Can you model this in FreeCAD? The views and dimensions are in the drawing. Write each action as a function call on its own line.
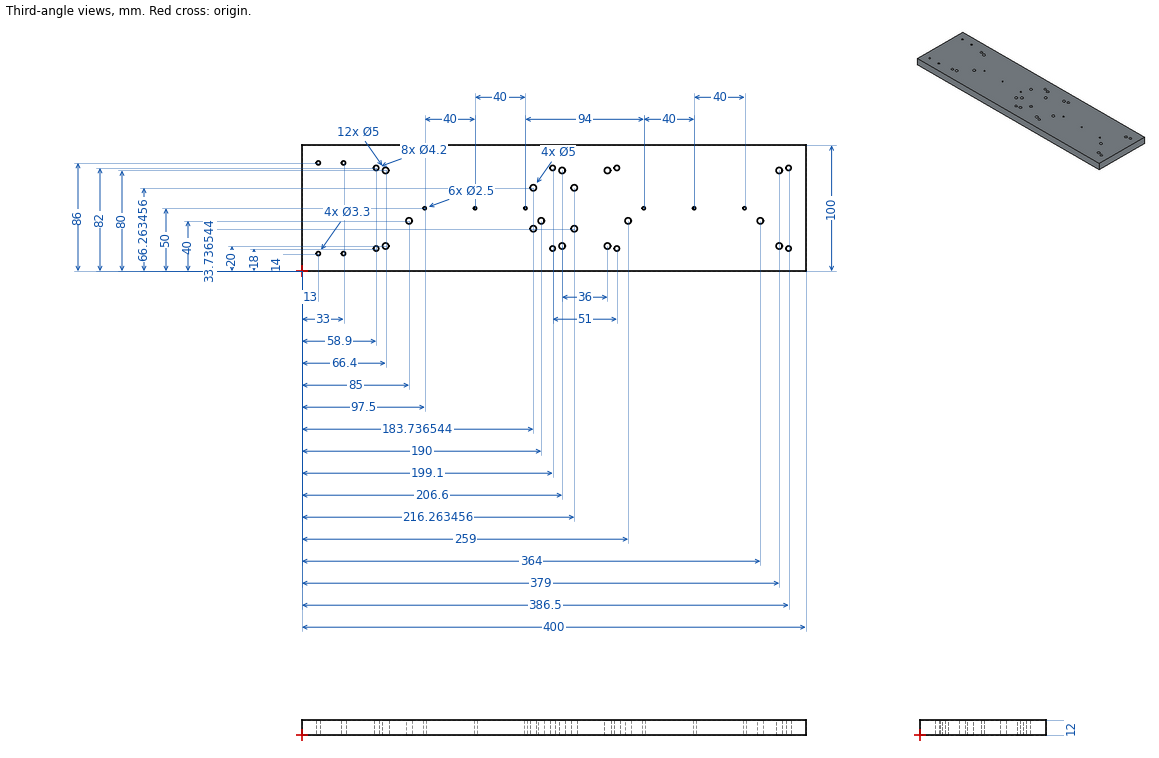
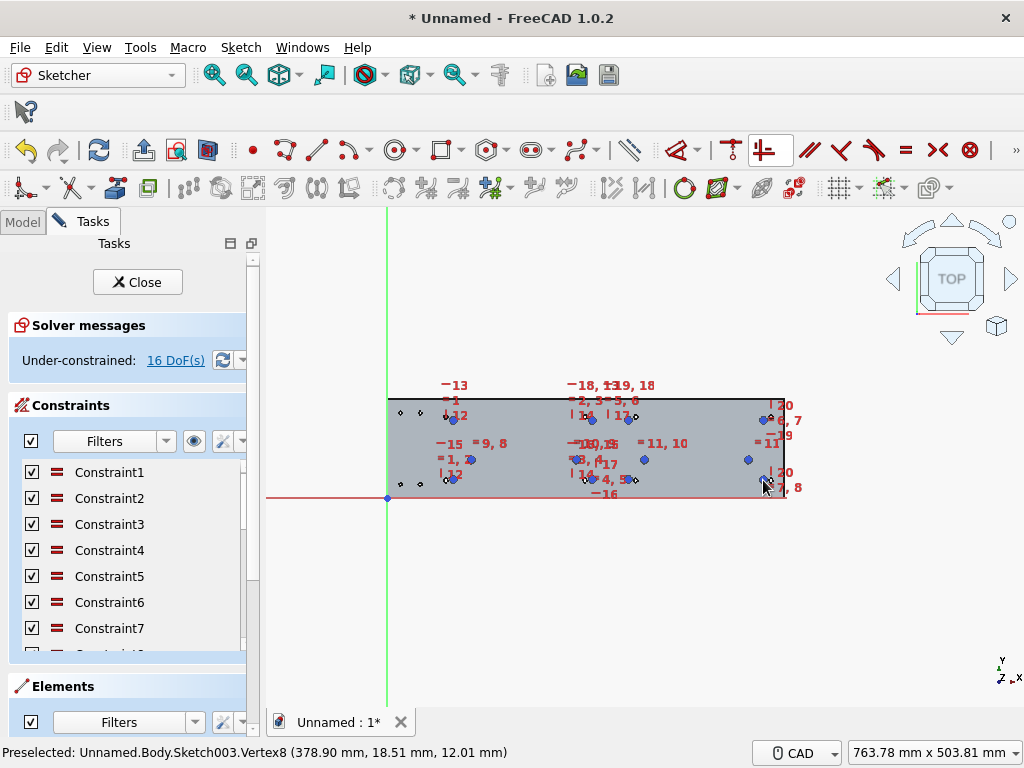
click(628, 479)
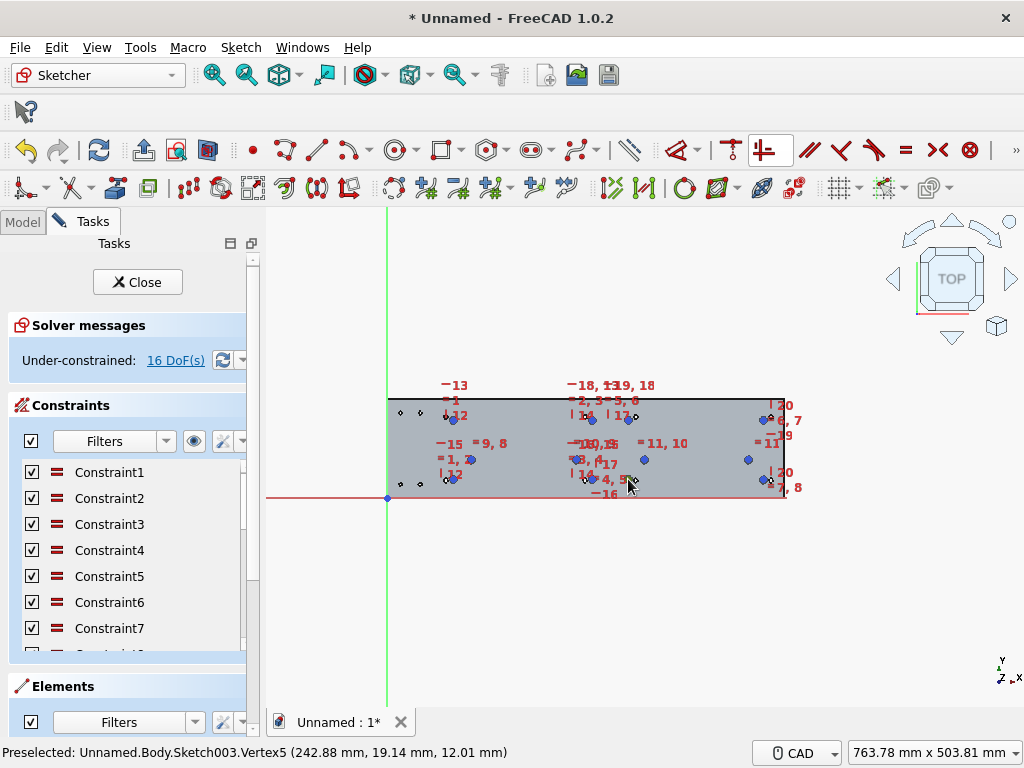
click(763, 480)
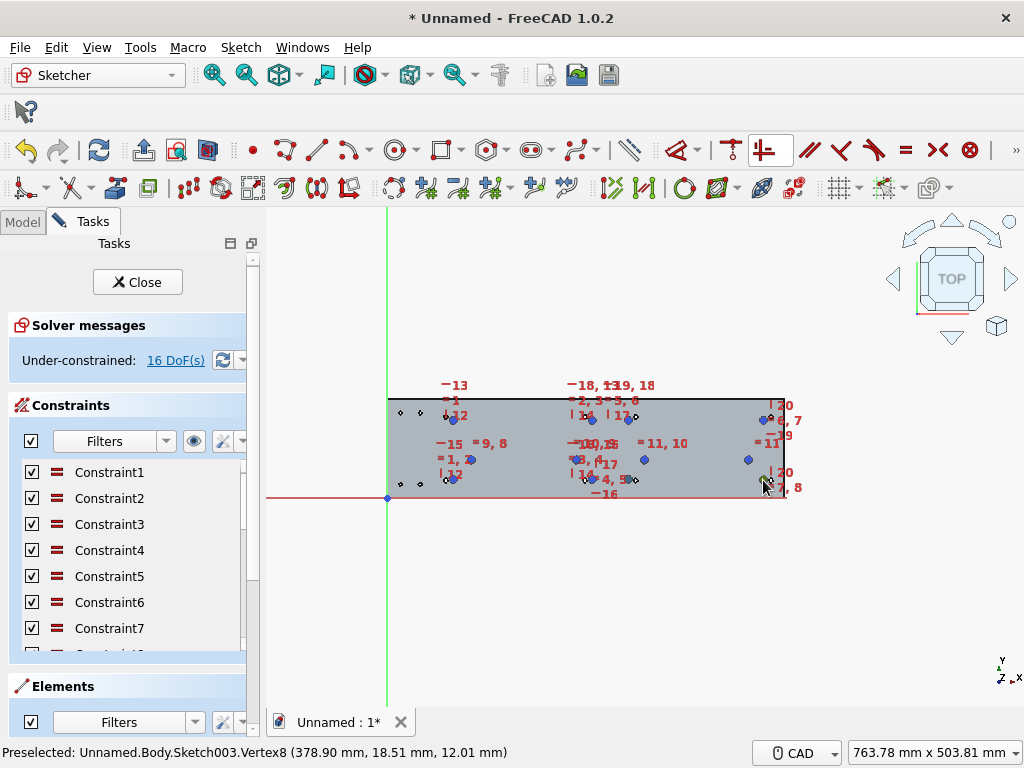
click(788, 150)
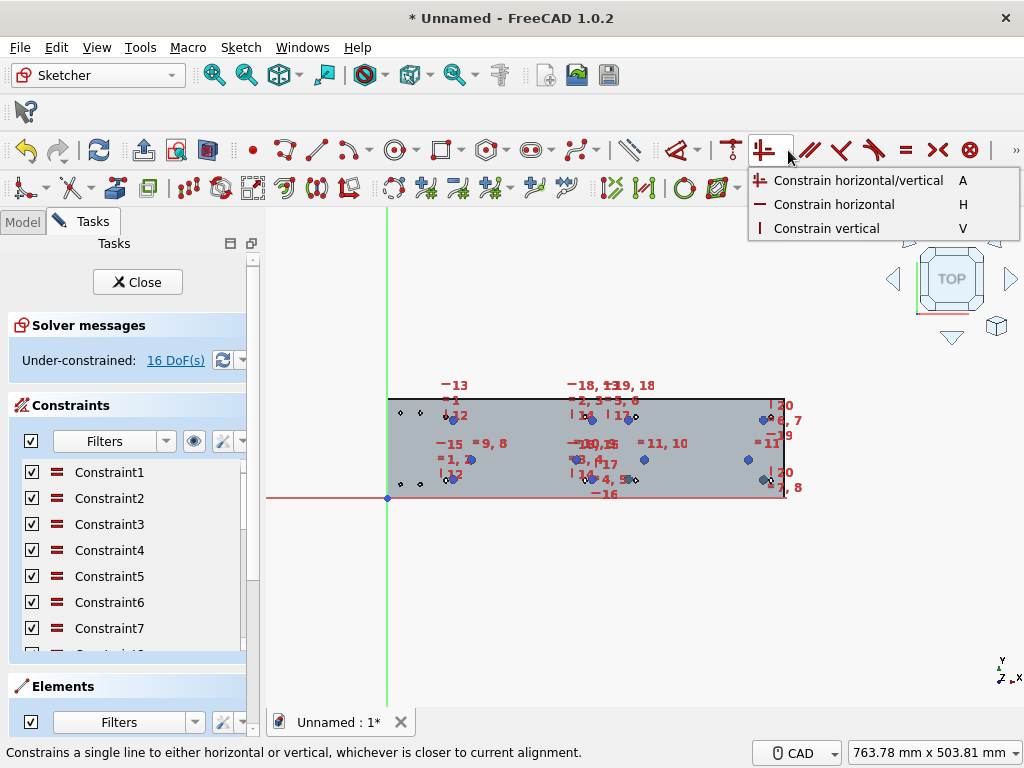
click(884, 204)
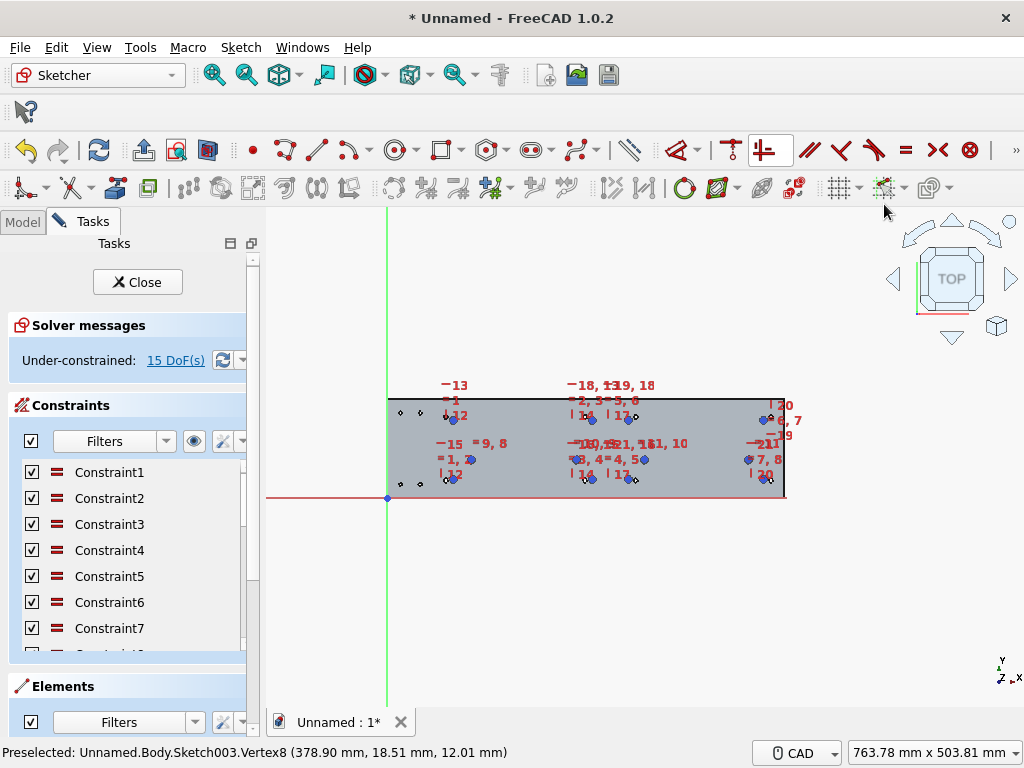
click(471, 460)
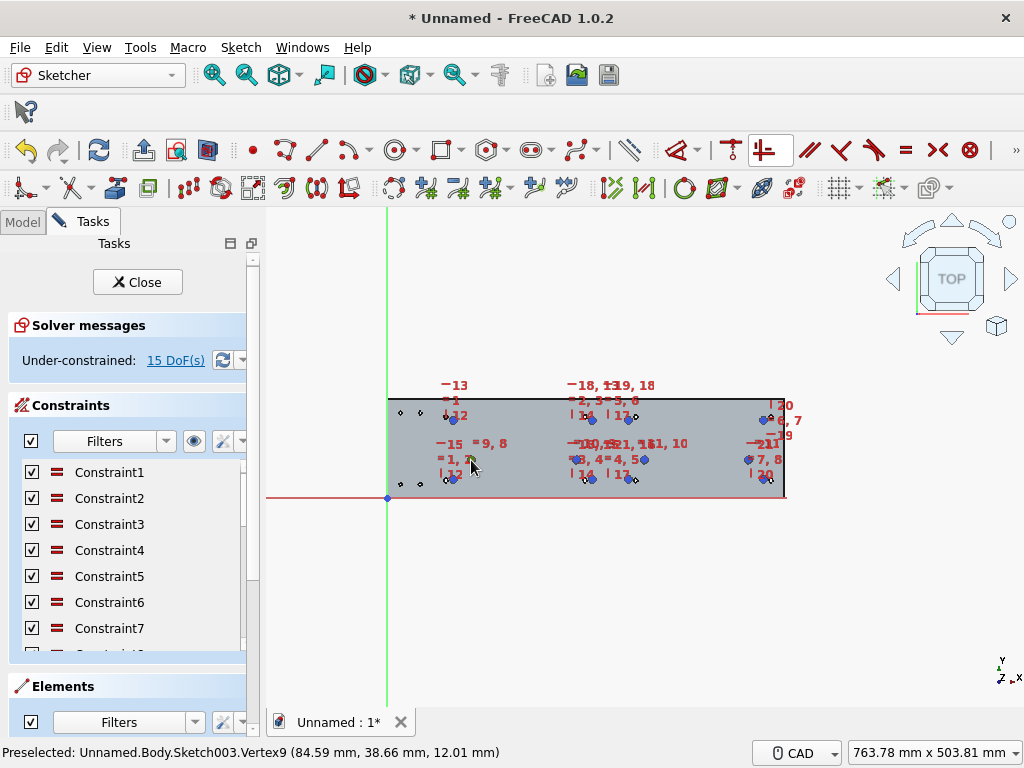
click(576, 460)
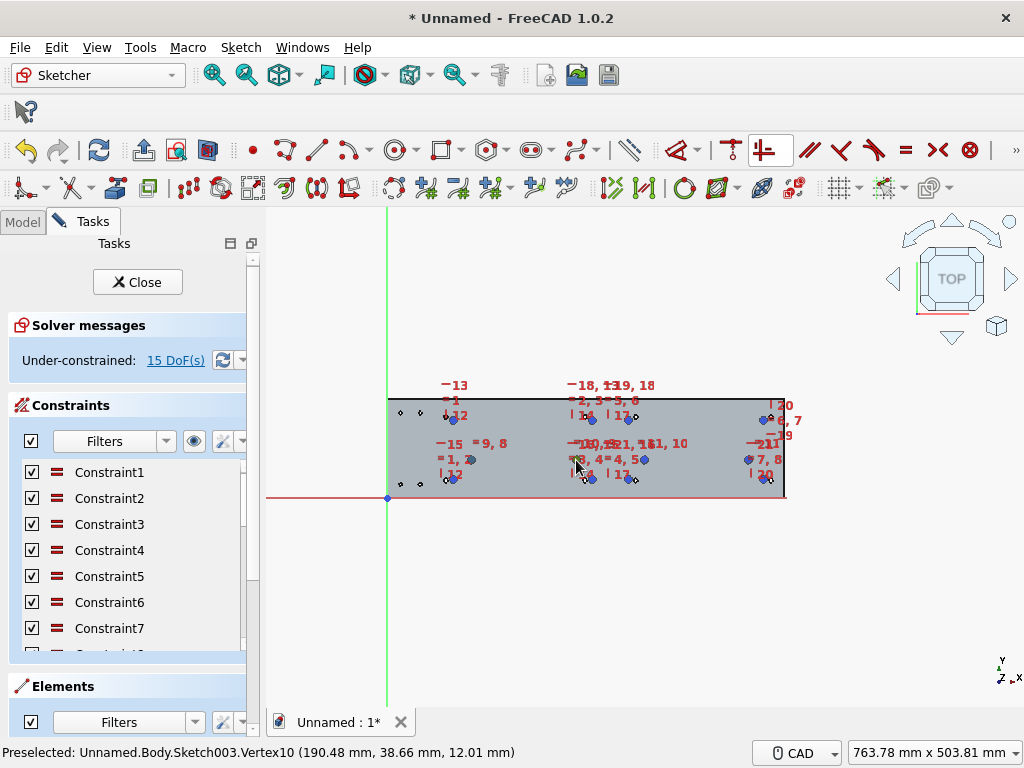
key(h)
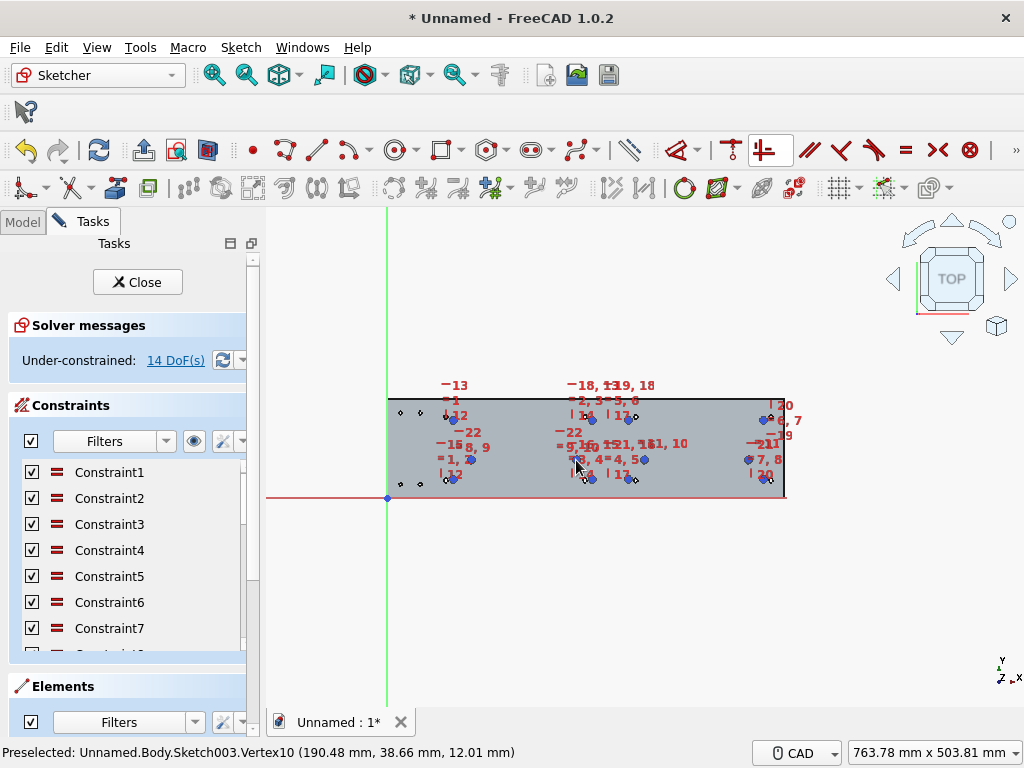
click(576, 460)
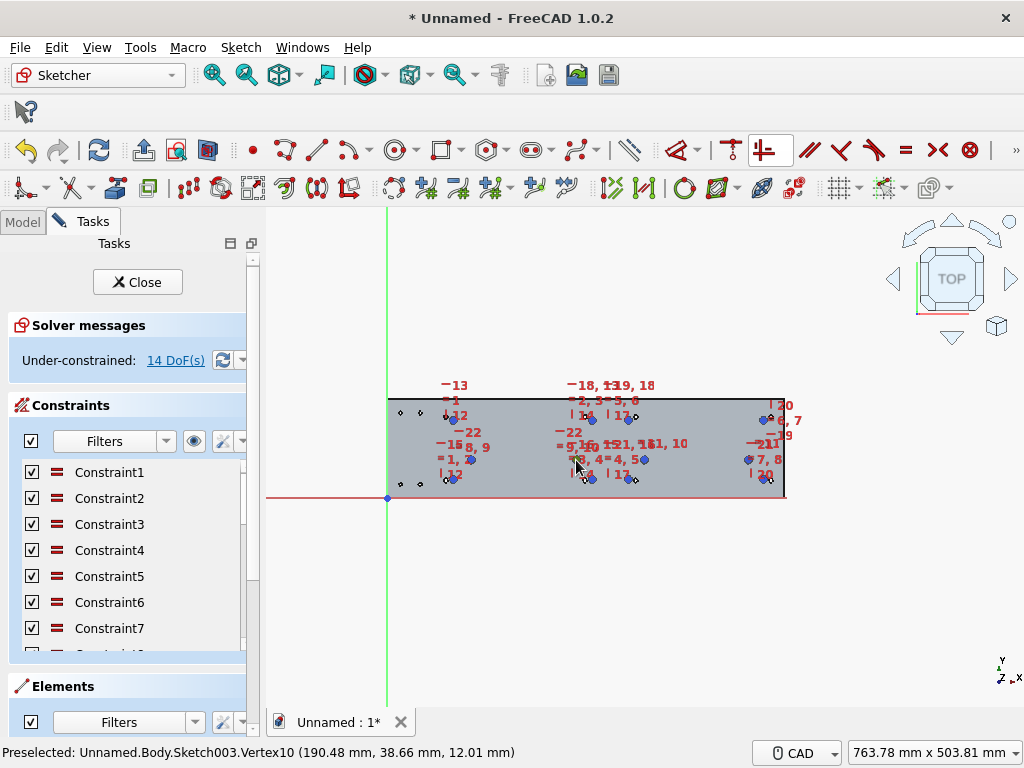
click(644, 460)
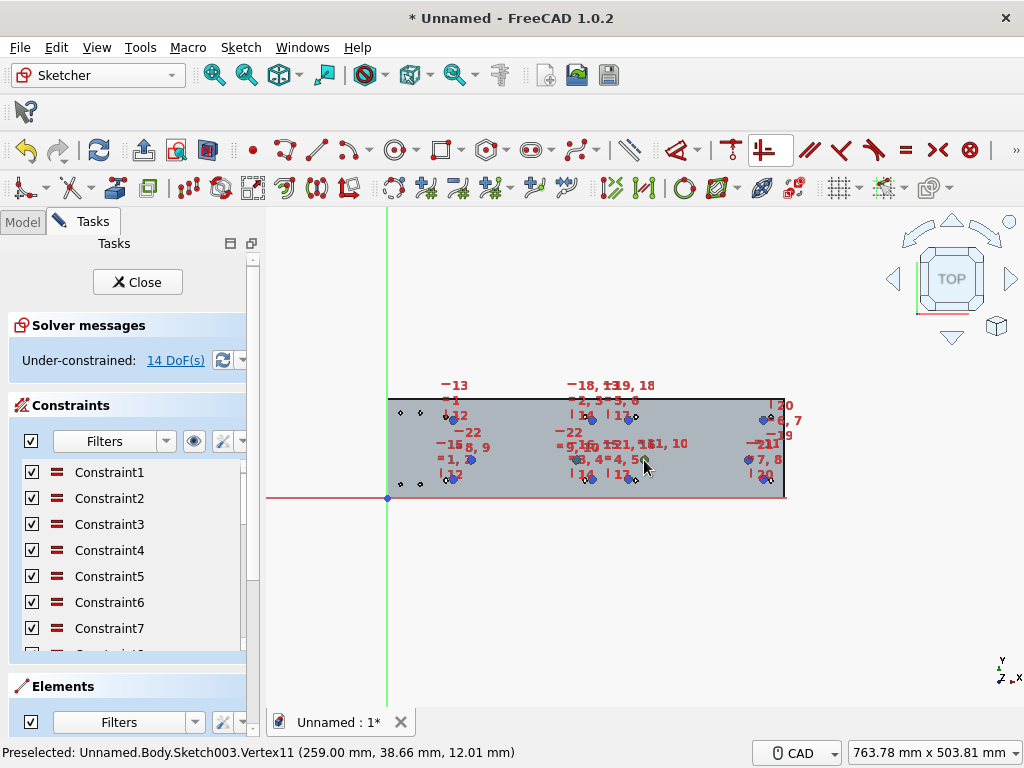
click(788, 150)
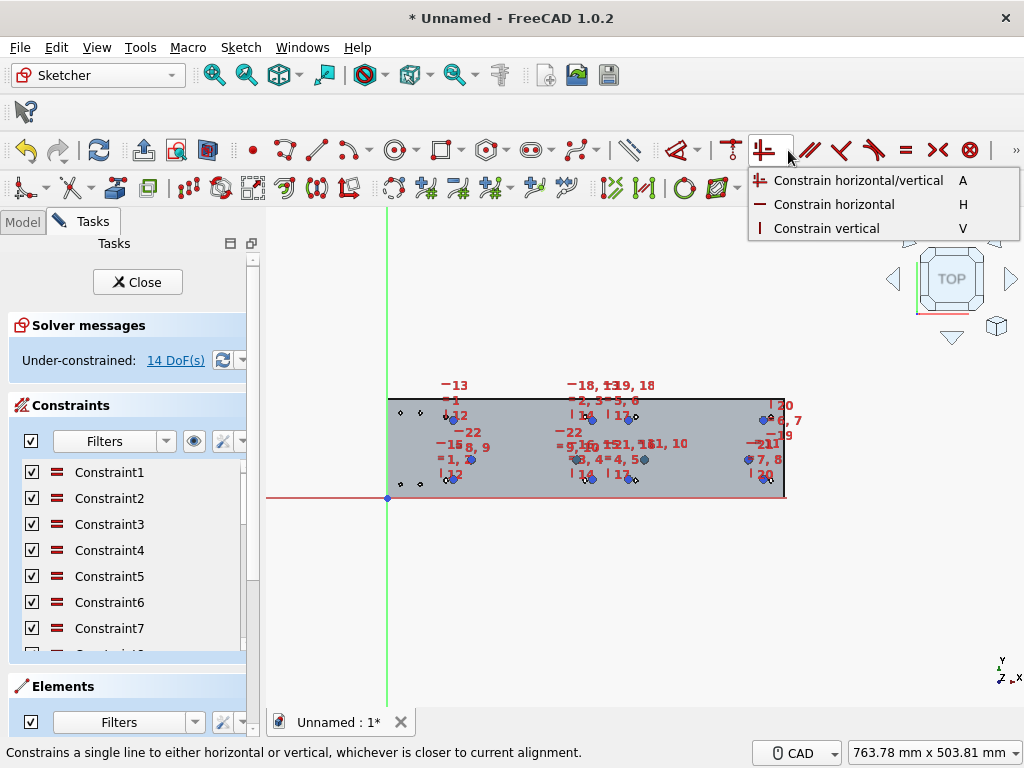
click(884, 204)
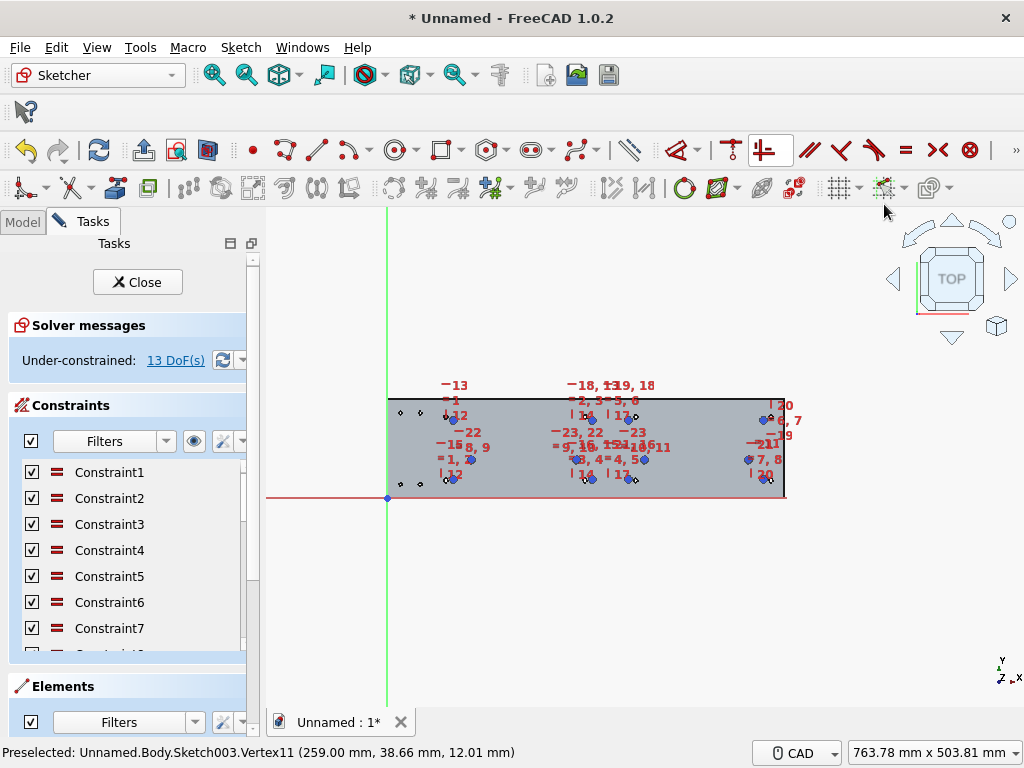
click(644, 460)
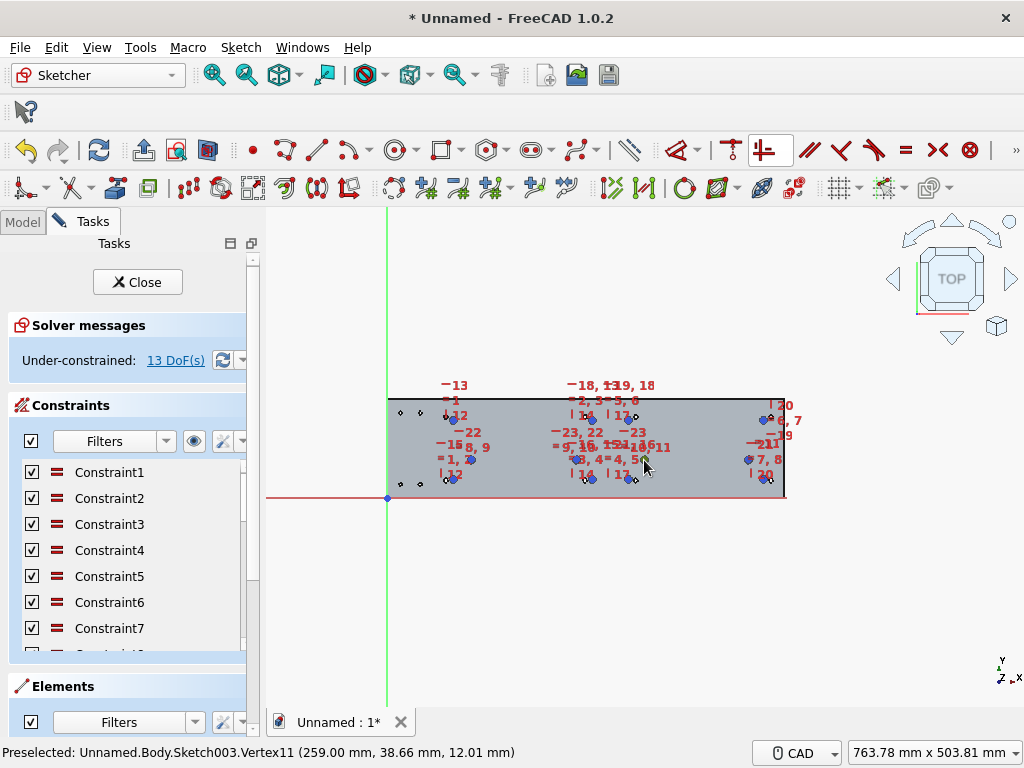
scroll(748, 460, up, 4)